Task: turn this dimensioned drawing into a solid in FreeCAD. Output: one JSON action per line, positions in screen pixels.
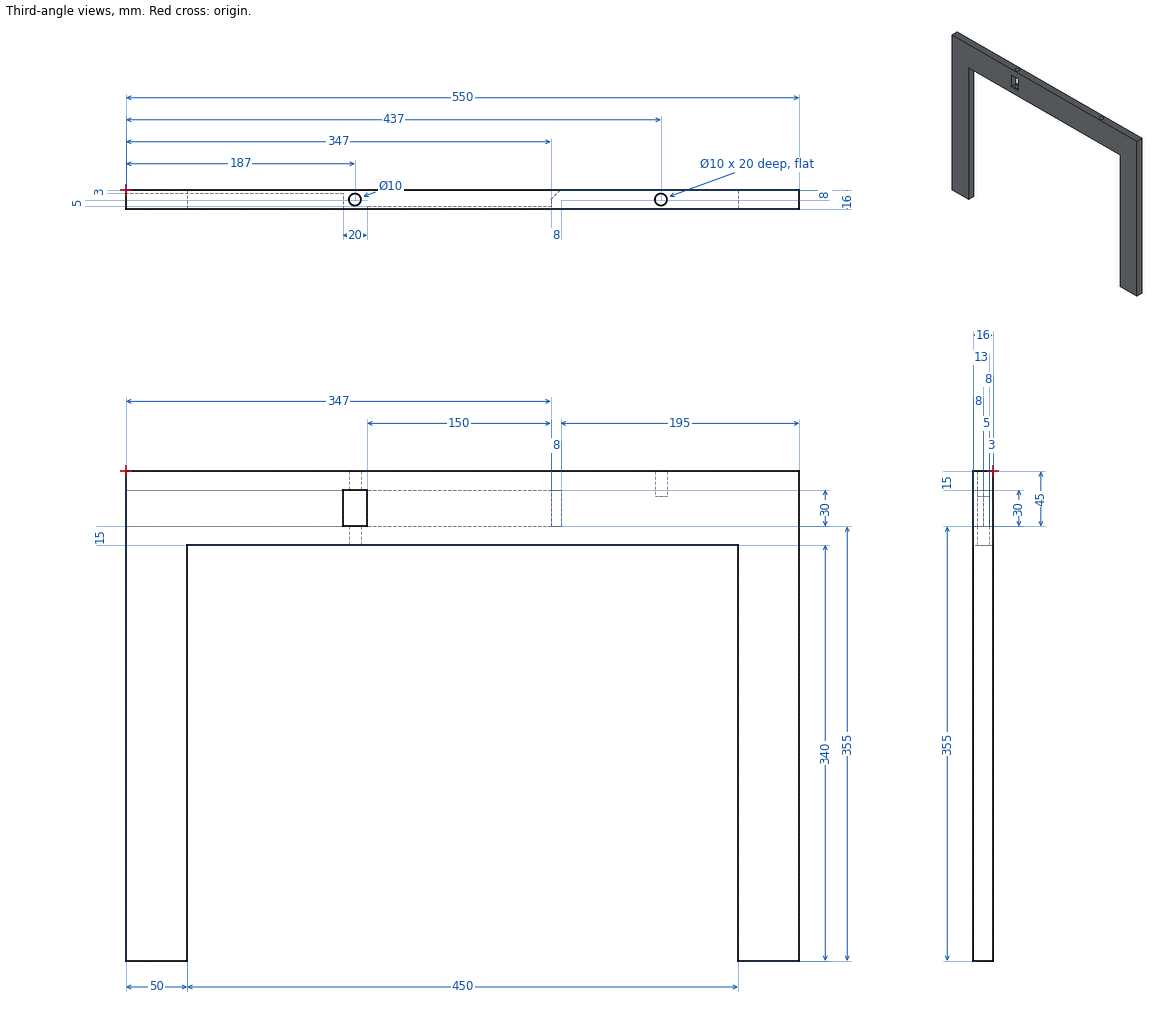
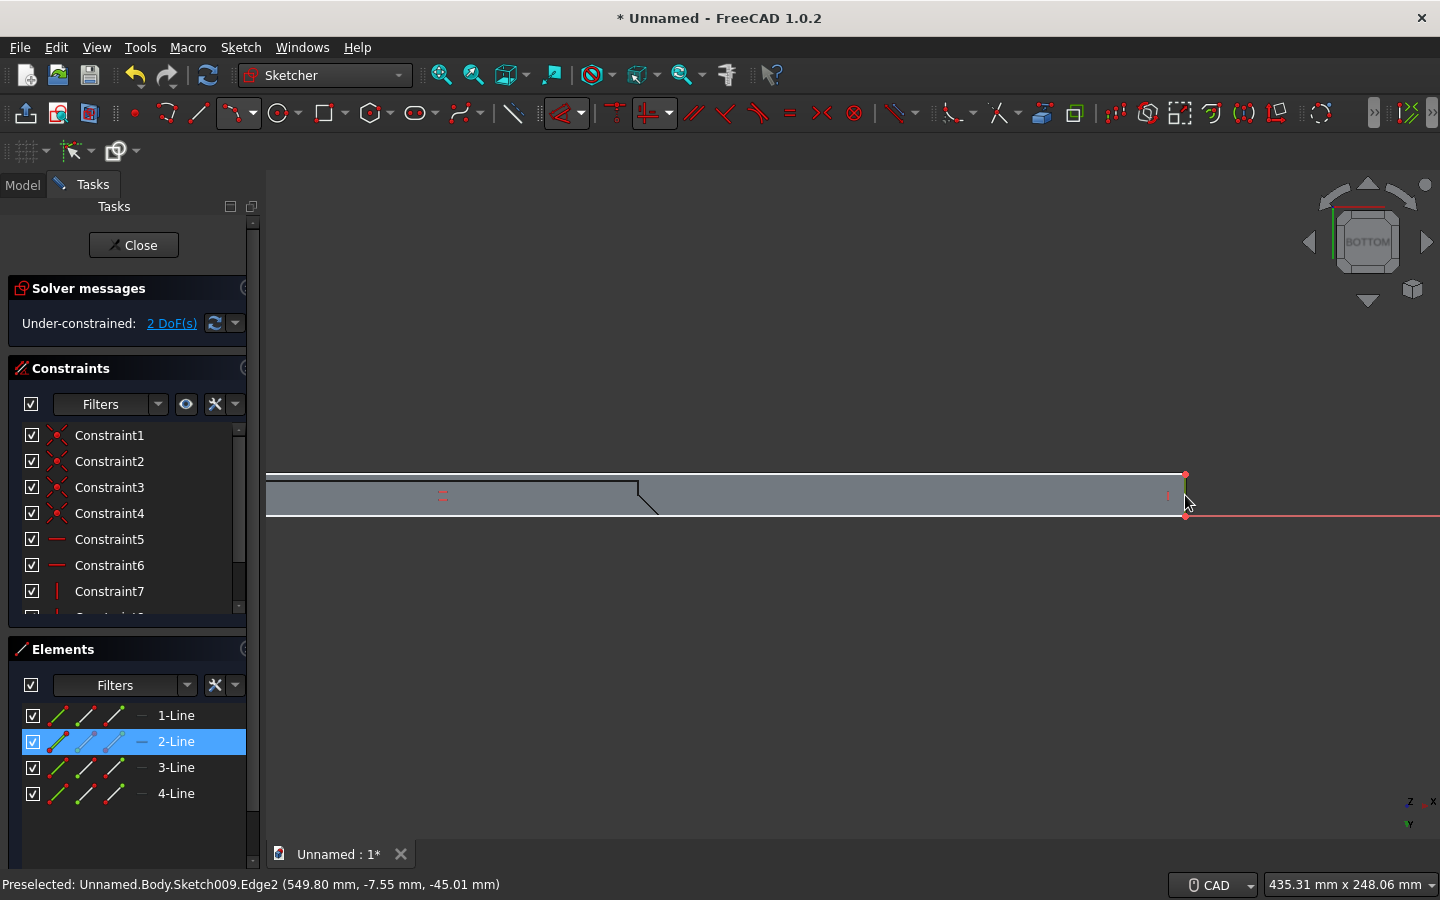
{"action": "key", "text": "i"}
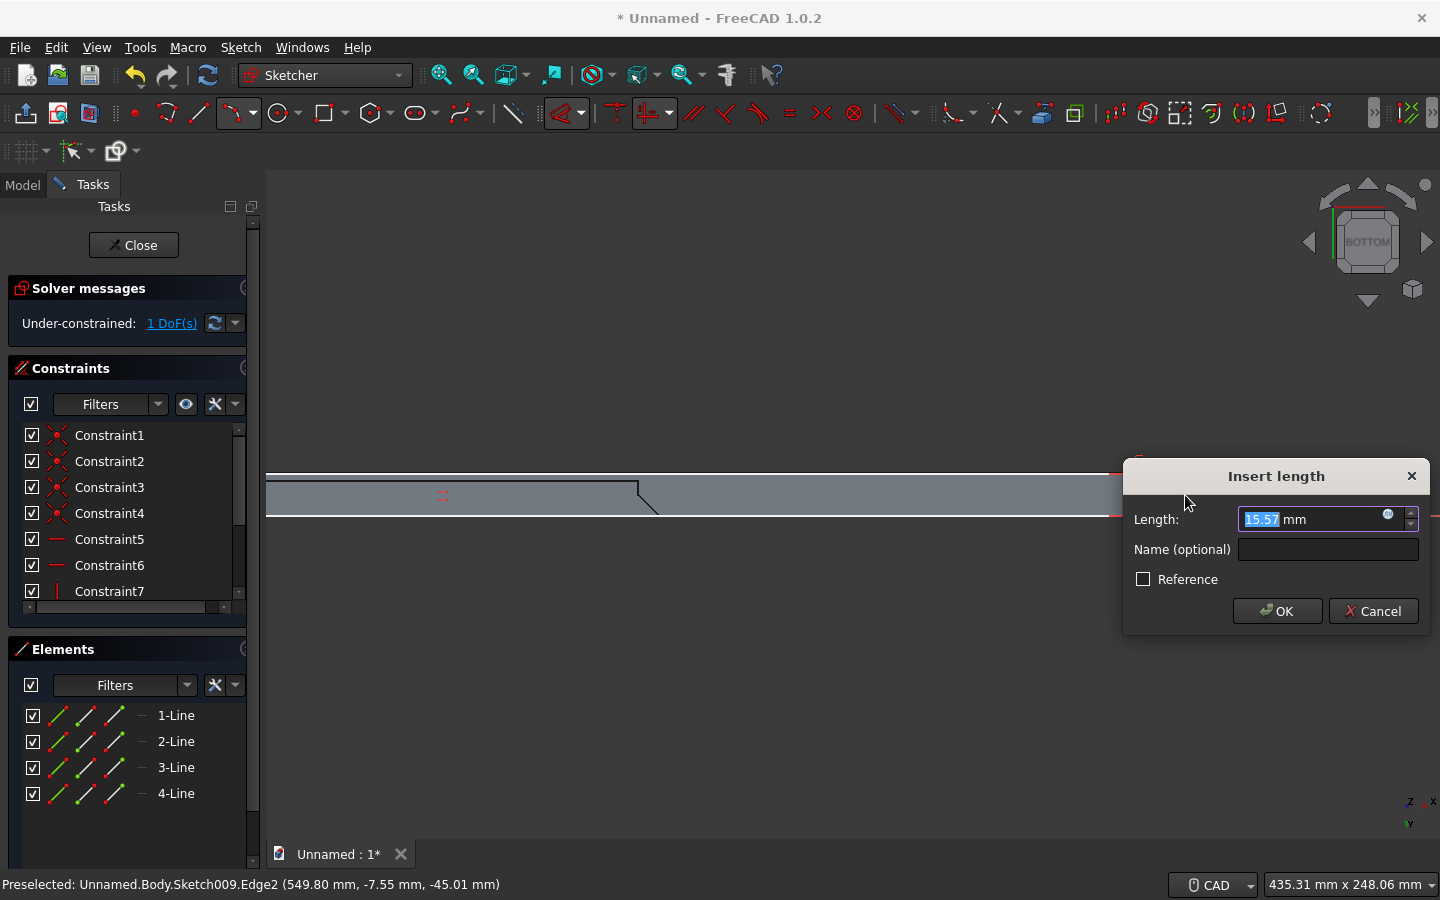
{"action": "type", "text": "16"}
{"action": "key", "text": "Return"}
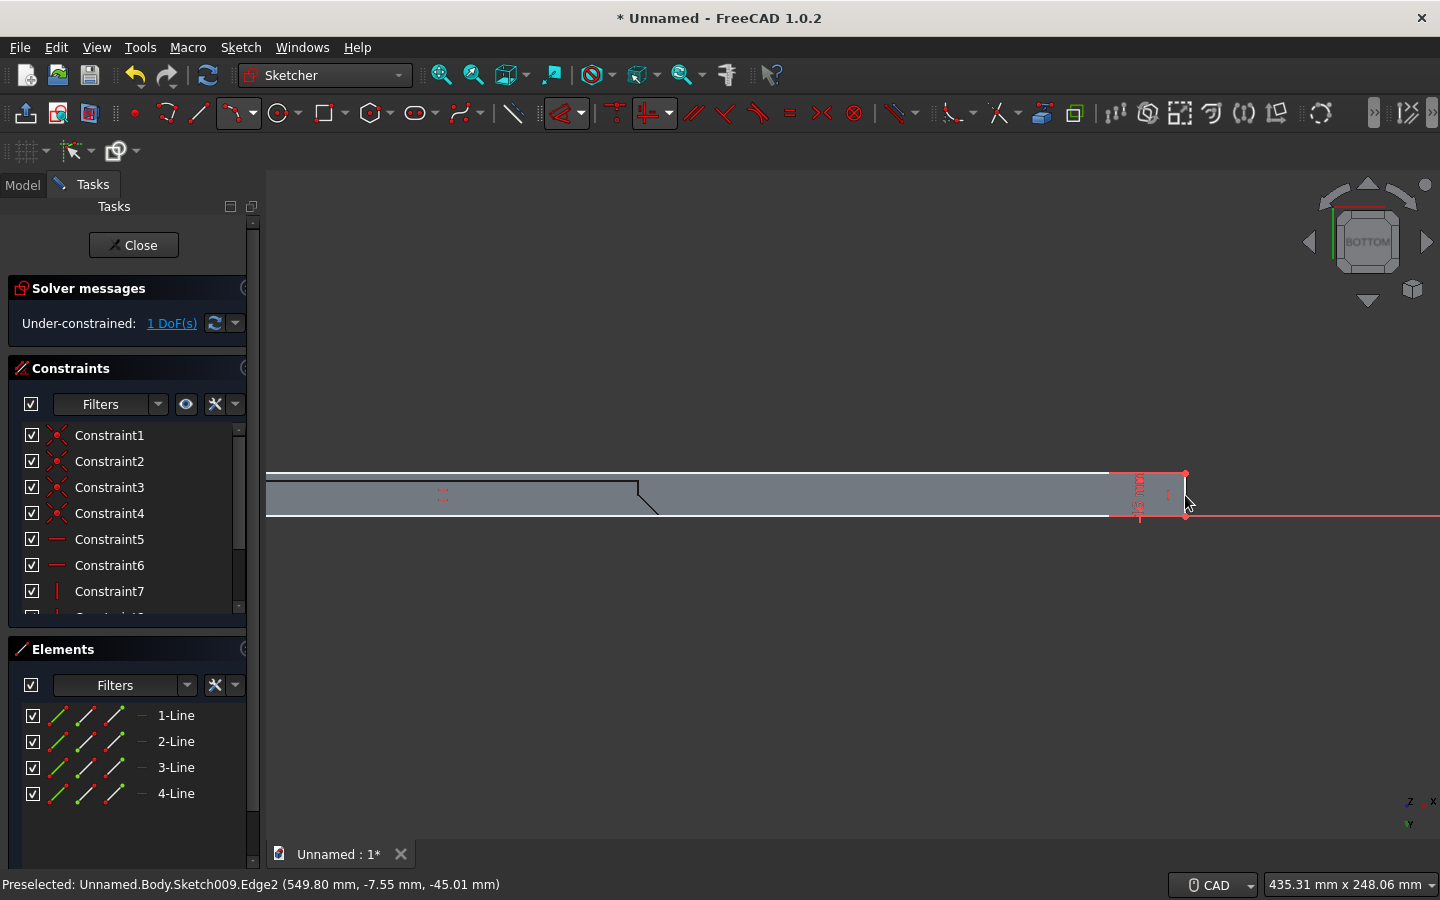
{"action": "left_click", "coordinate": [740, 516]}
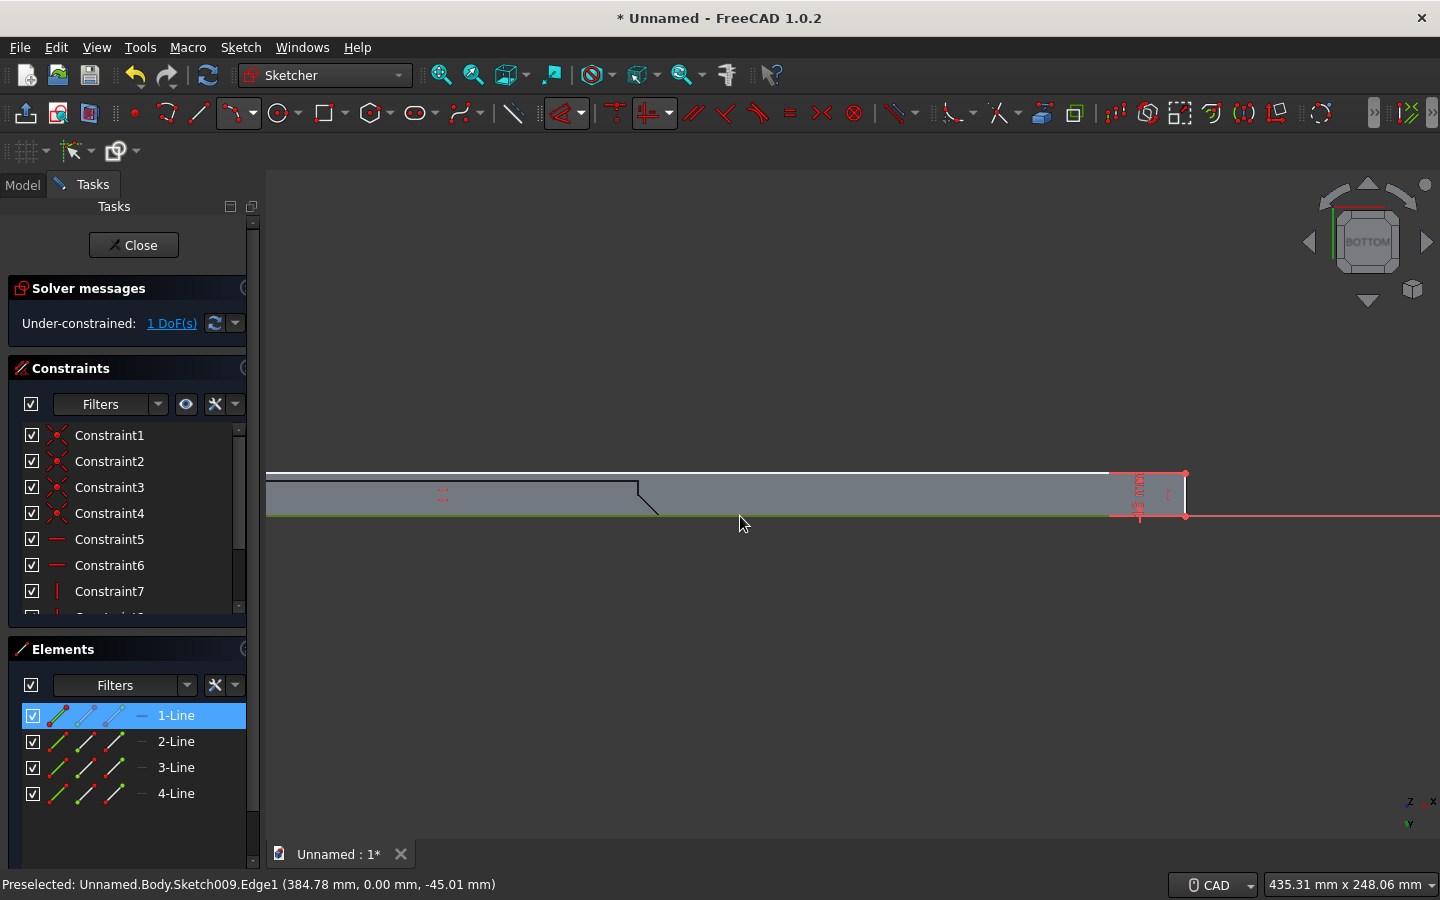
{"action": "key", "text": "l"}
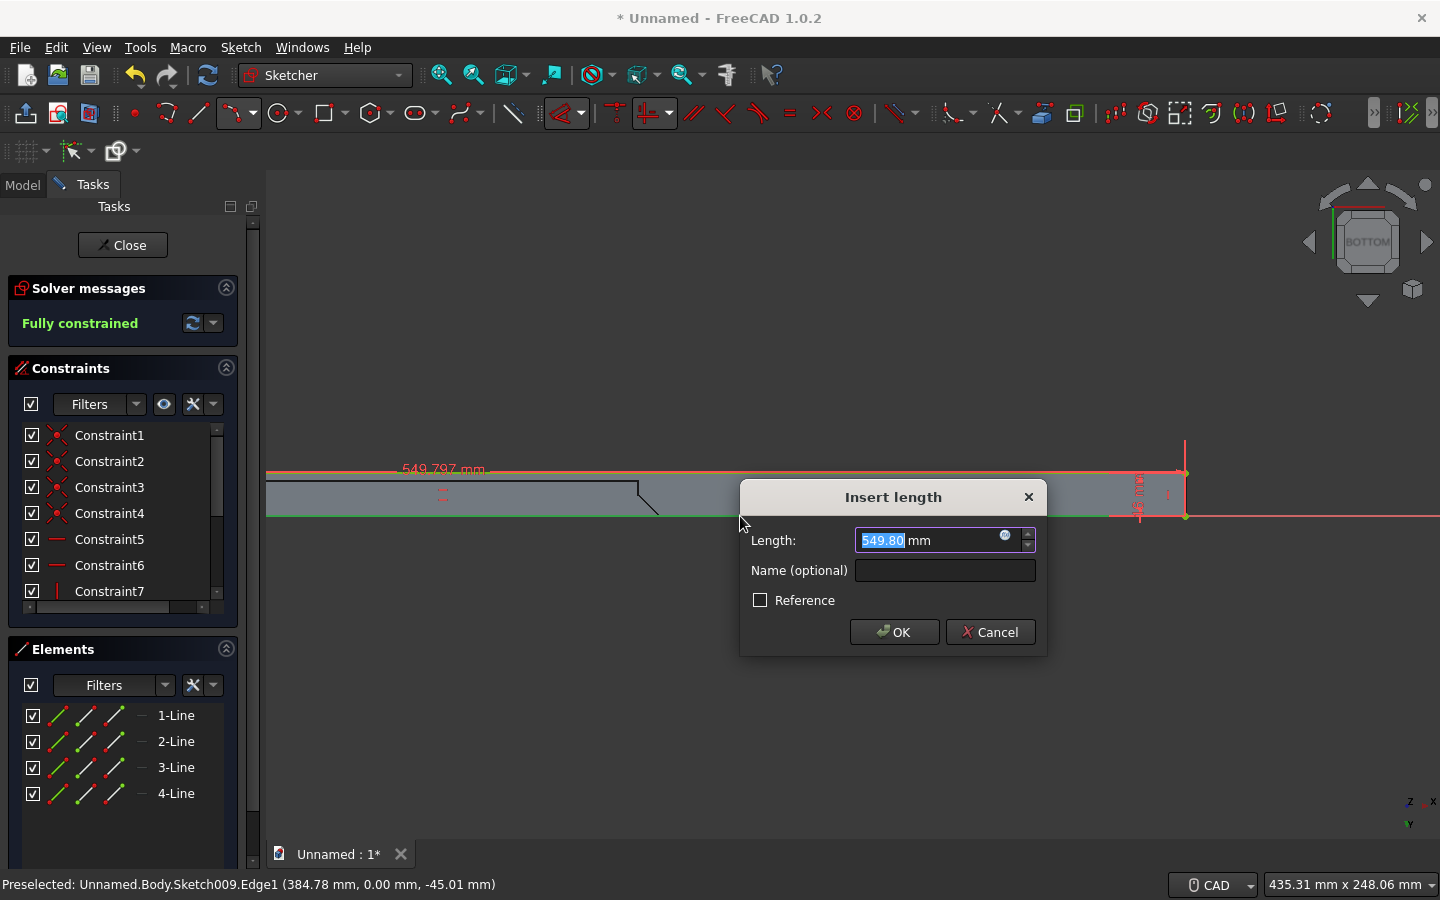
{"action": "type", "text": "550"}
{"action": "key", "text": "Return"}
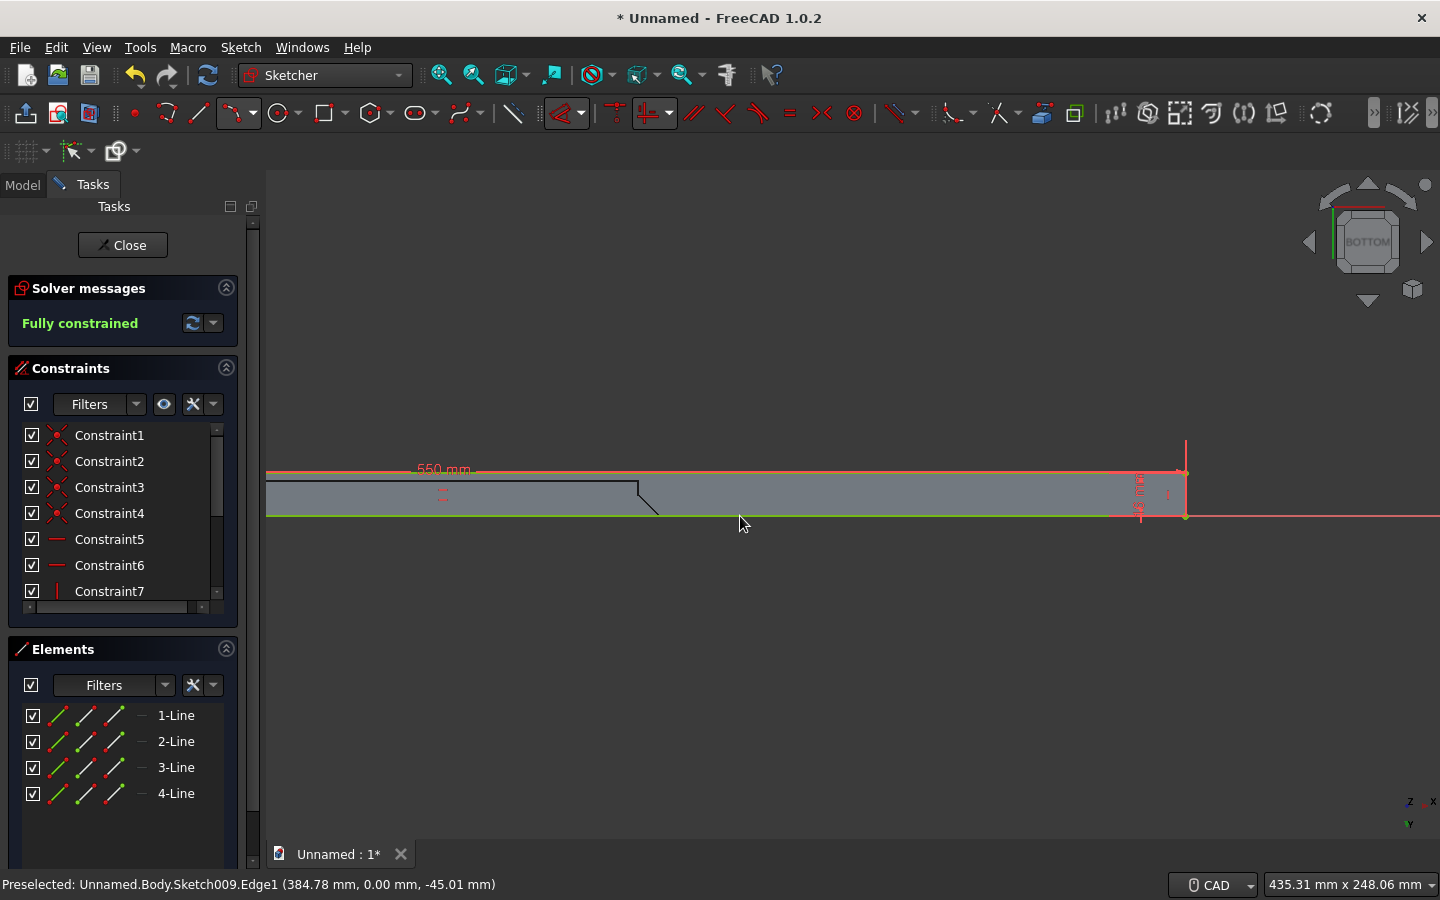
{"action": "left_click", "coordinate": [123, 245]}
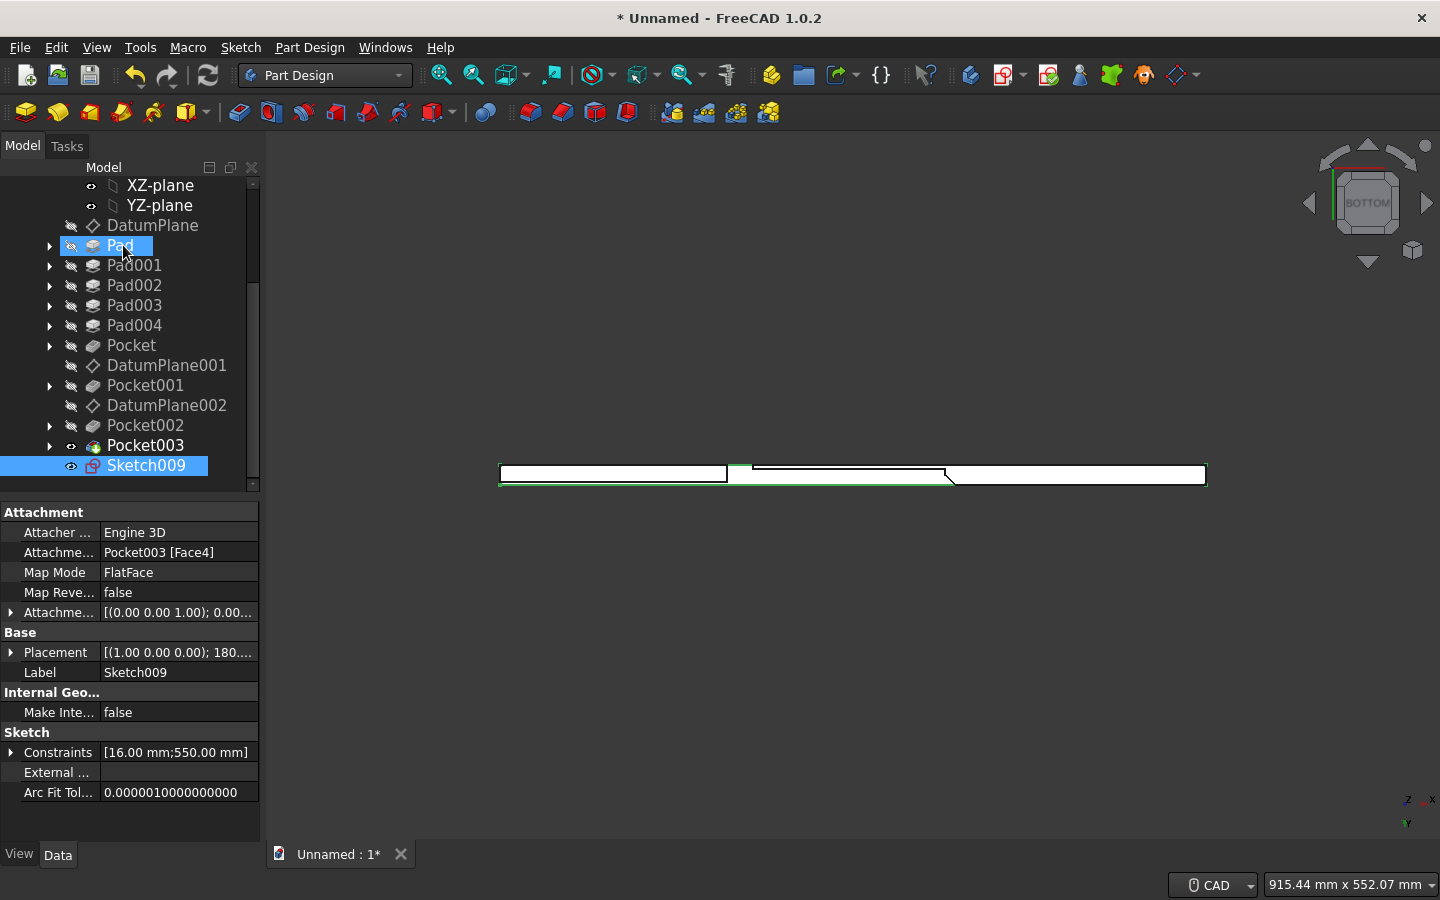
{"action": "left_click", "coordinate": [26, 112]}